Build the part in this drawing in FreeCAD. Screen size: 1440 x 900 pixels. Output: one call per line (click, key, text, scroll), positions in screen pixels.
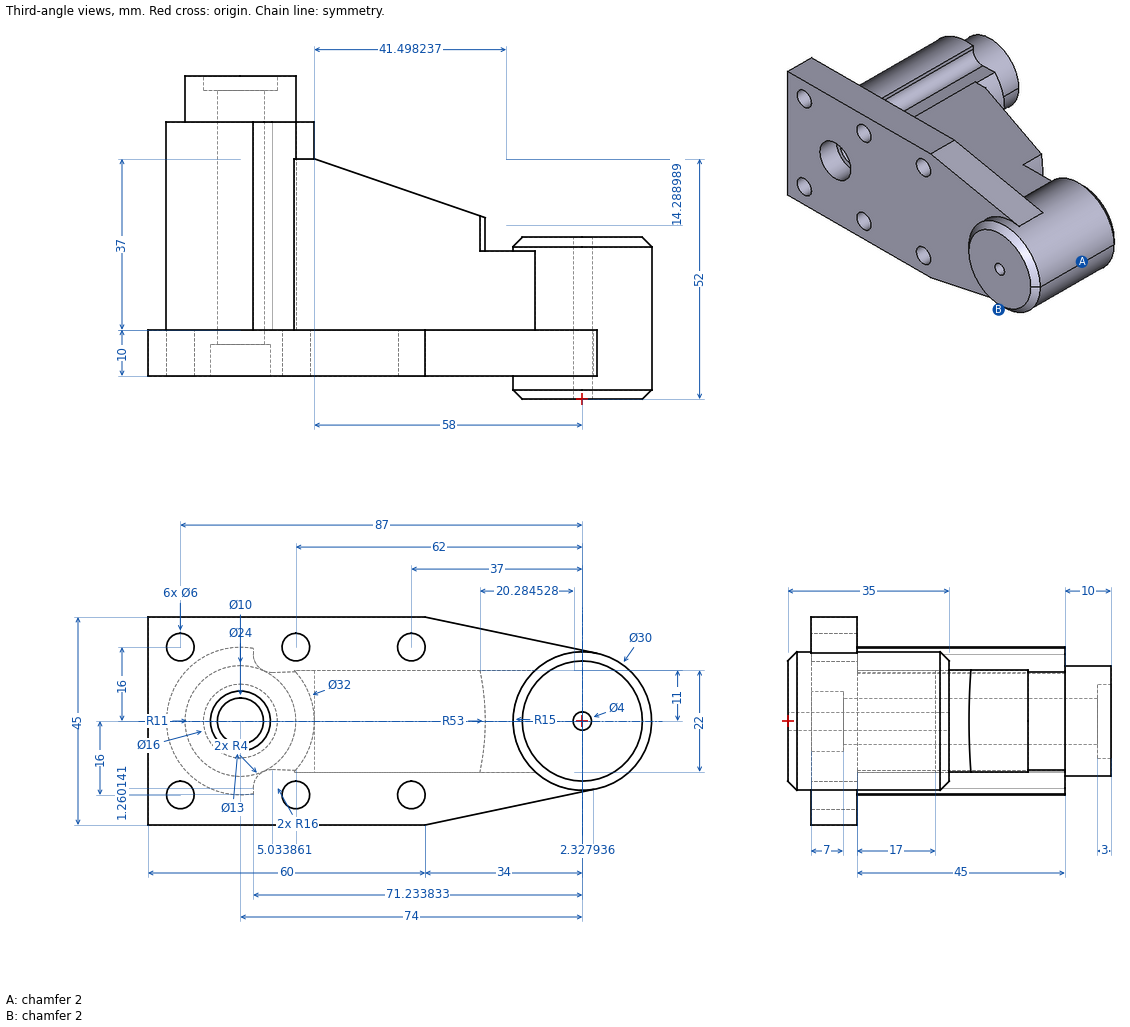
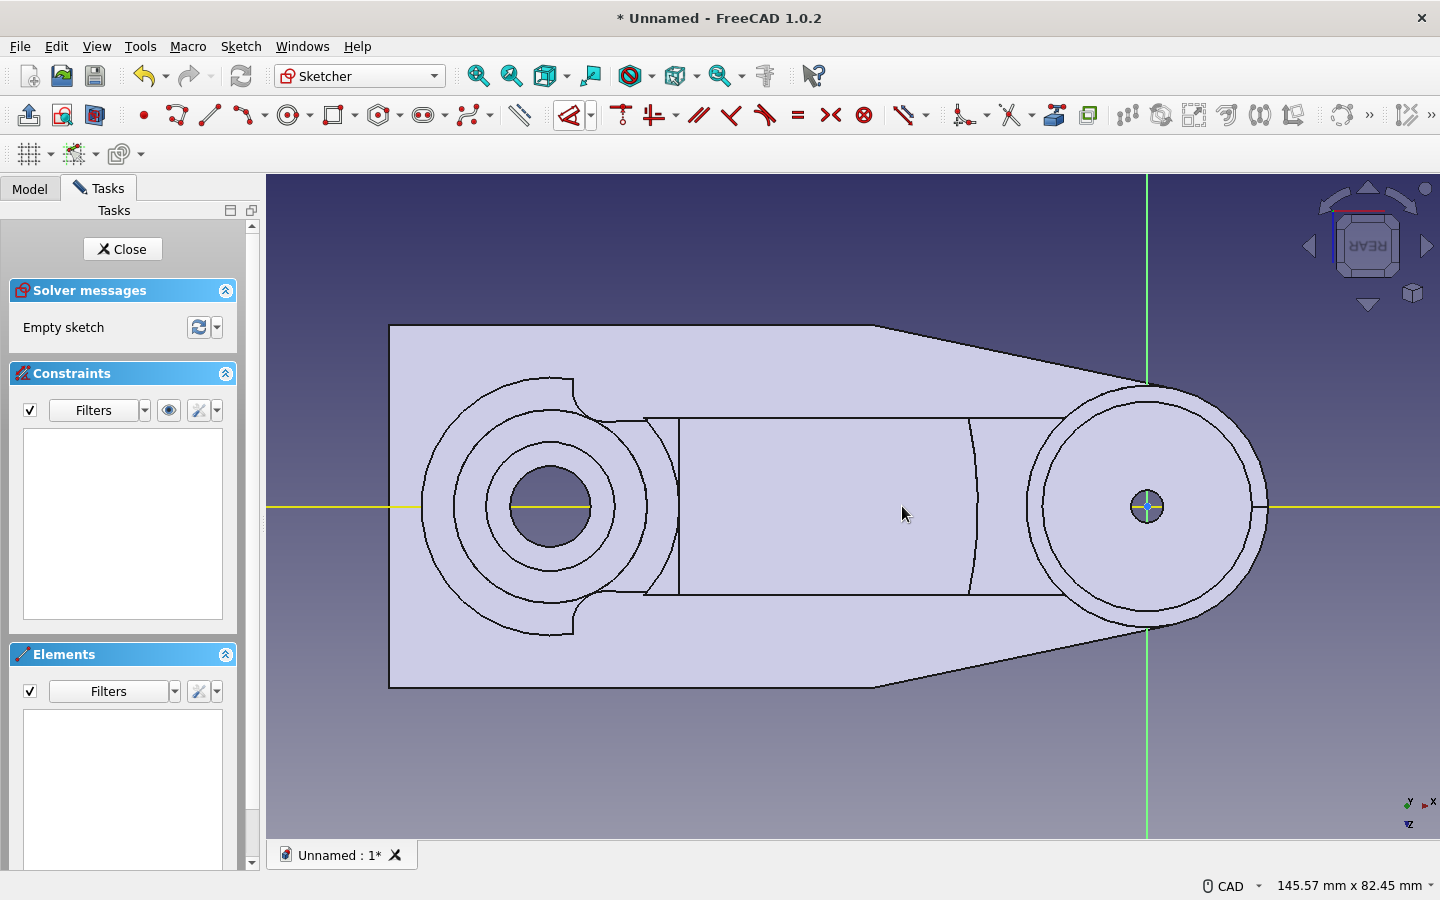
click(288, 116)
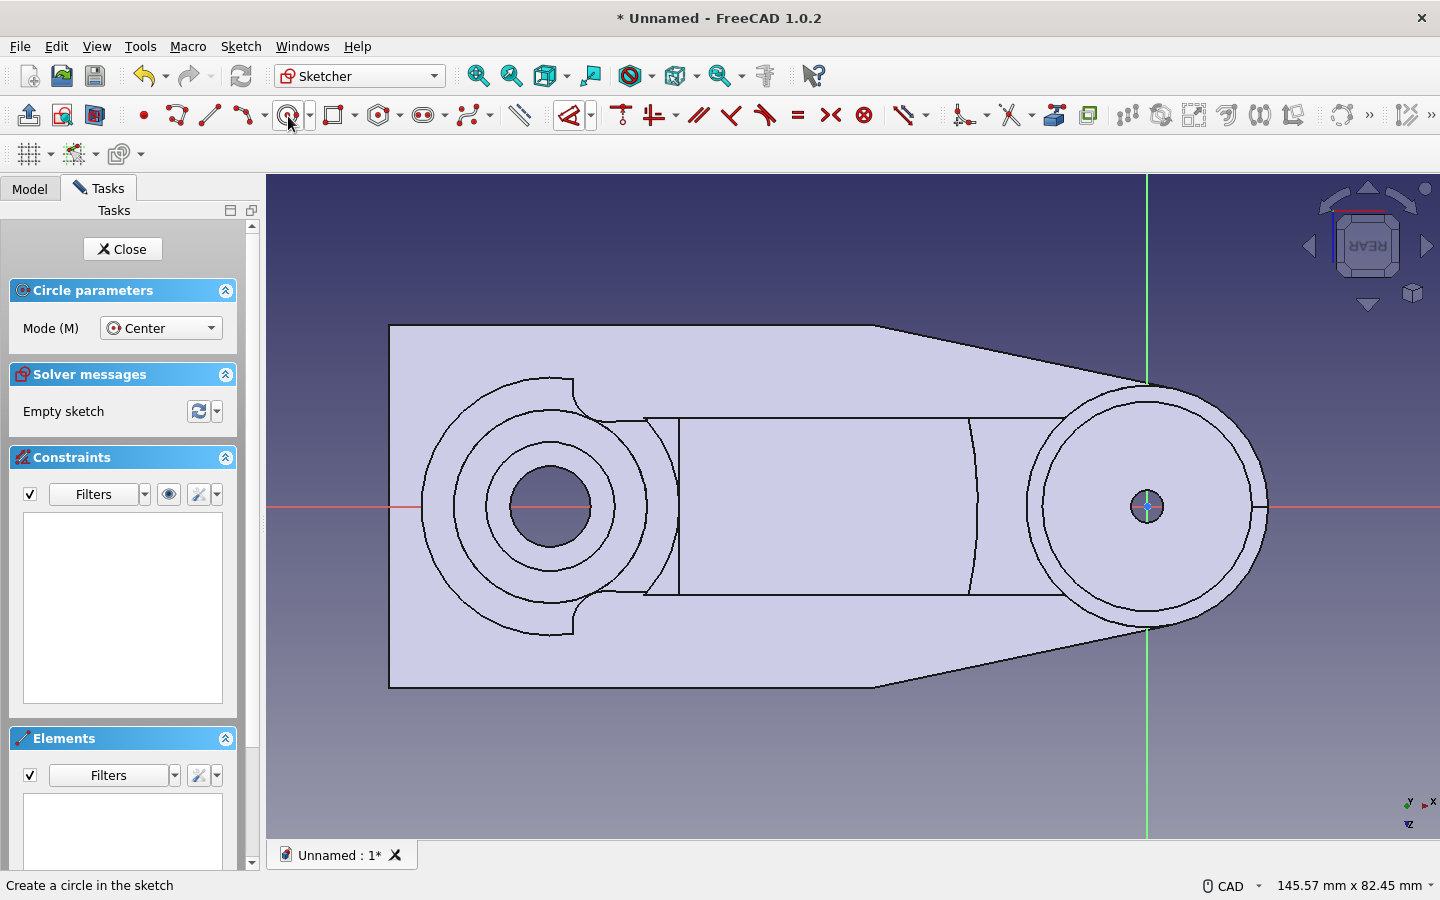
click(446, 636)
click(463, 618)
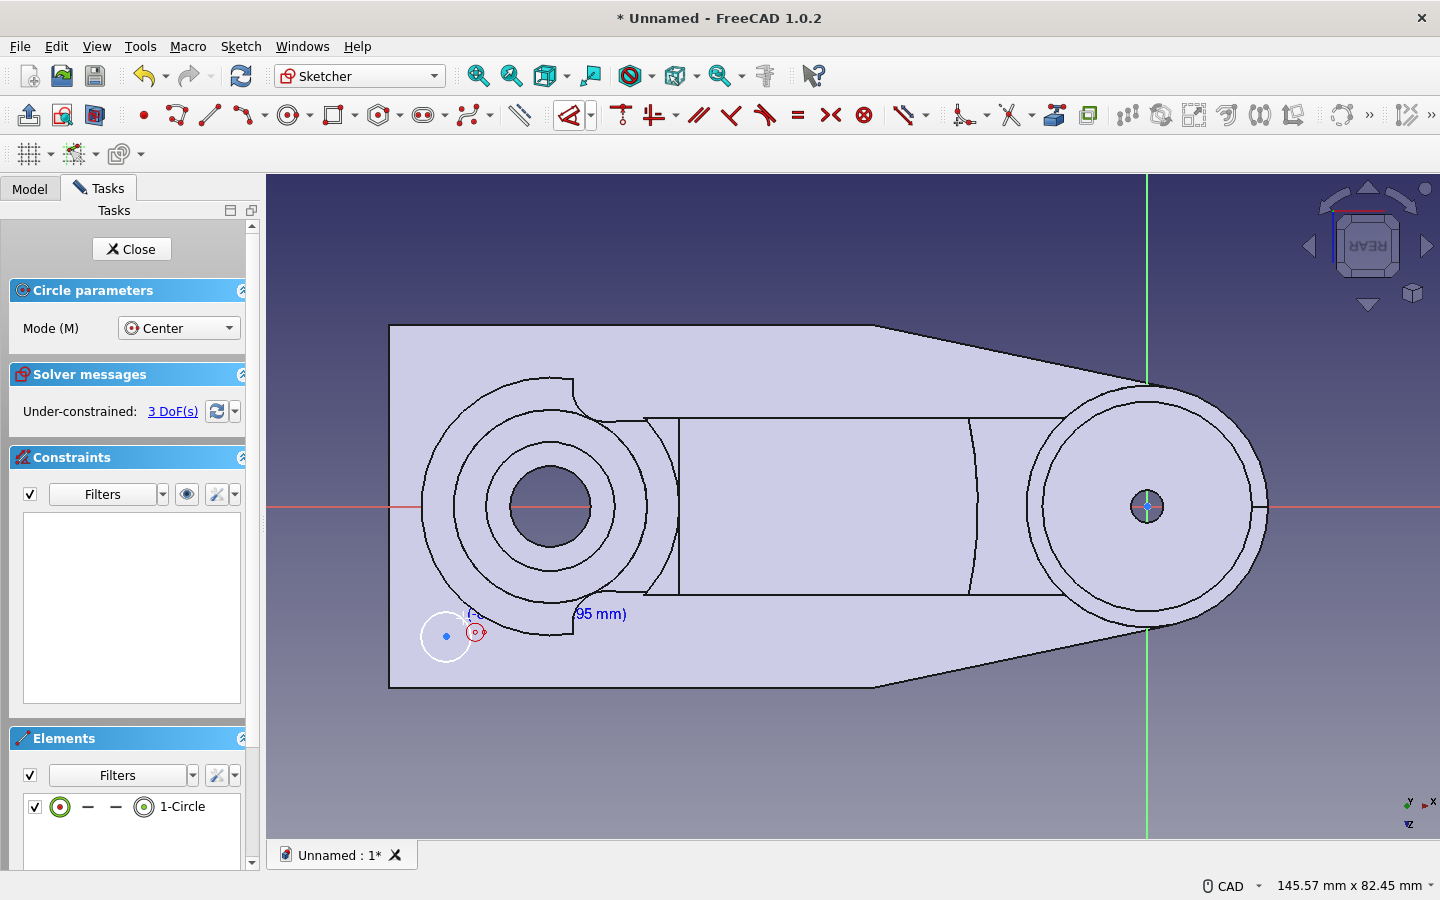
click(647, 636)
click(664, 618)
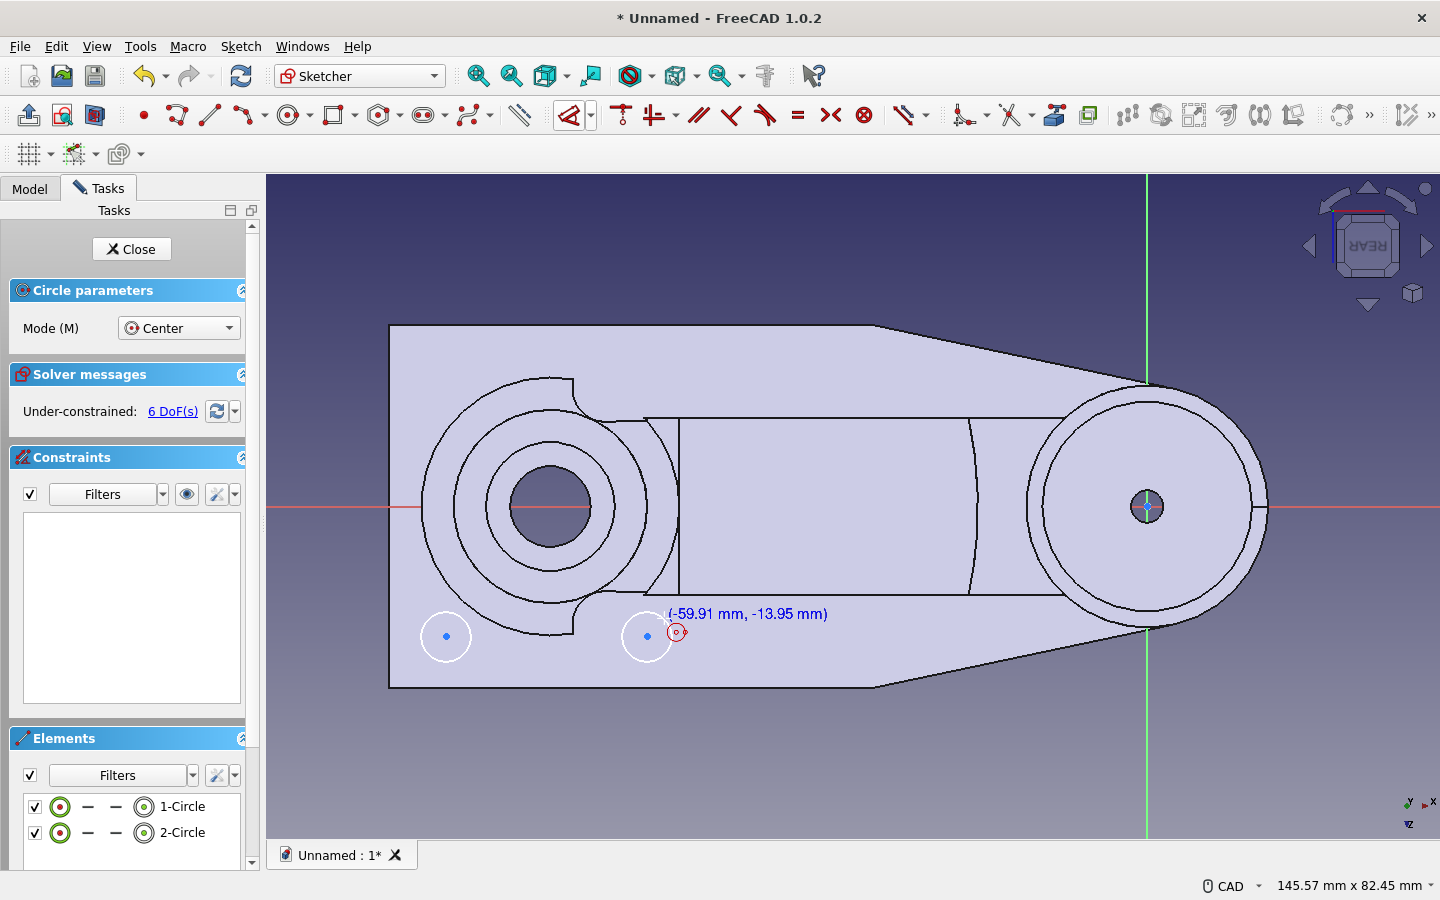
click(849, 636)
click(866, 618)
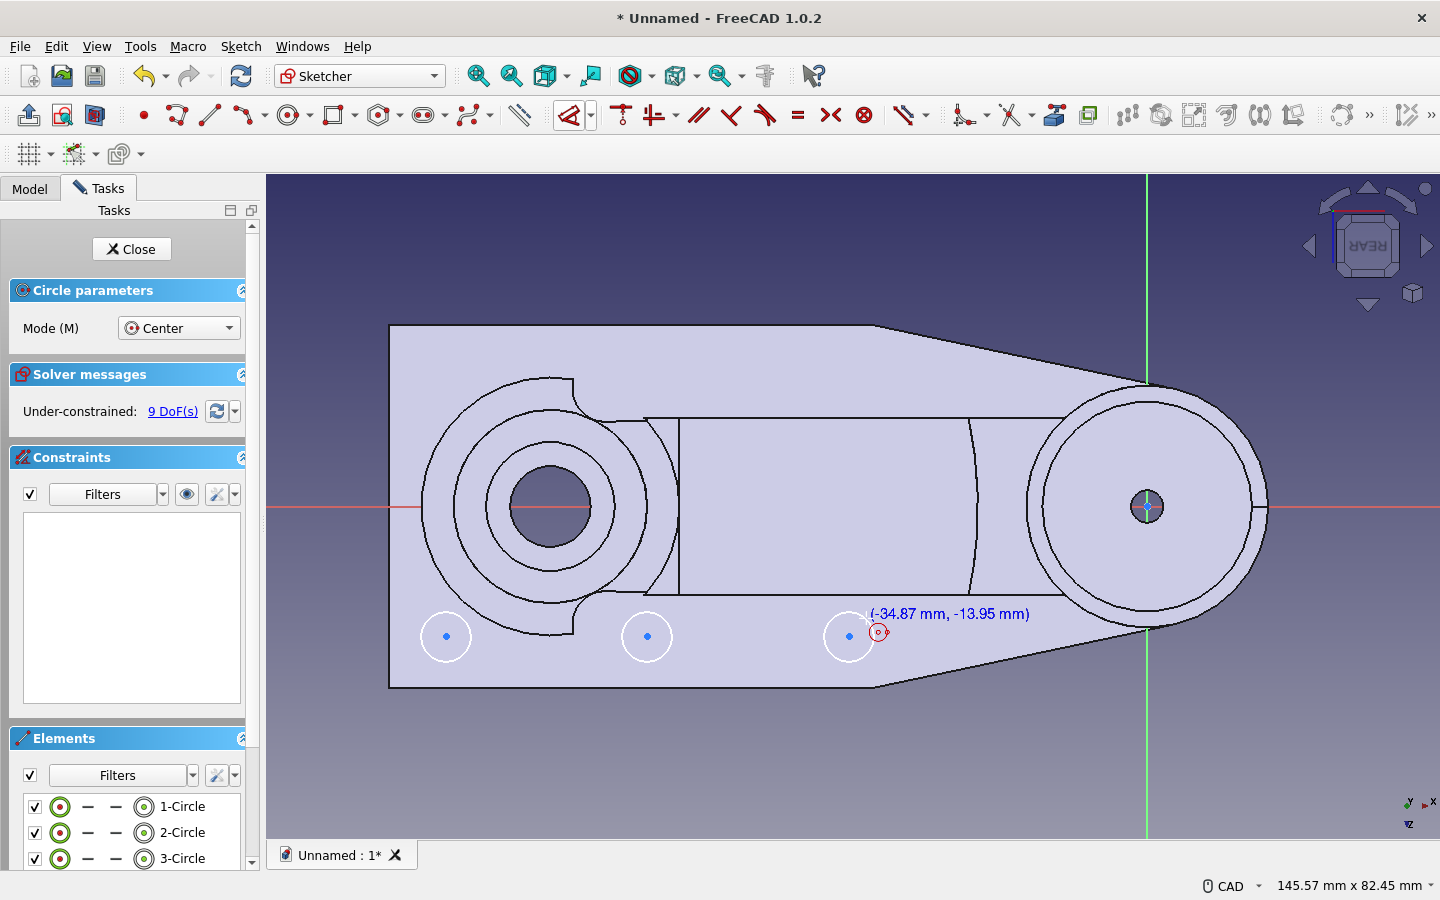
click(446, 377)
click(463, 360)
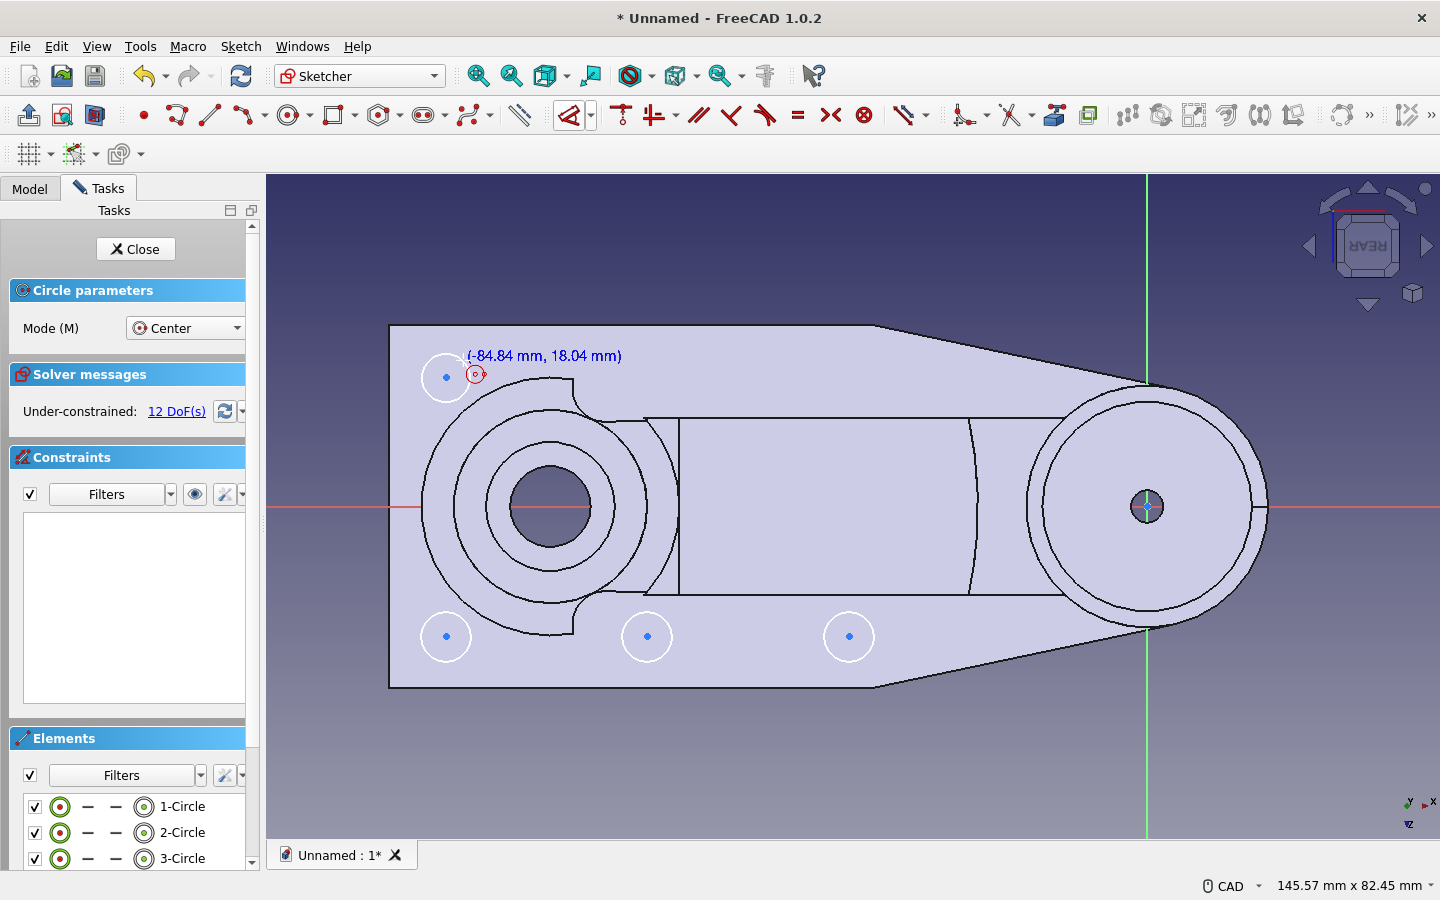
click(849, 377)
click(866, 360)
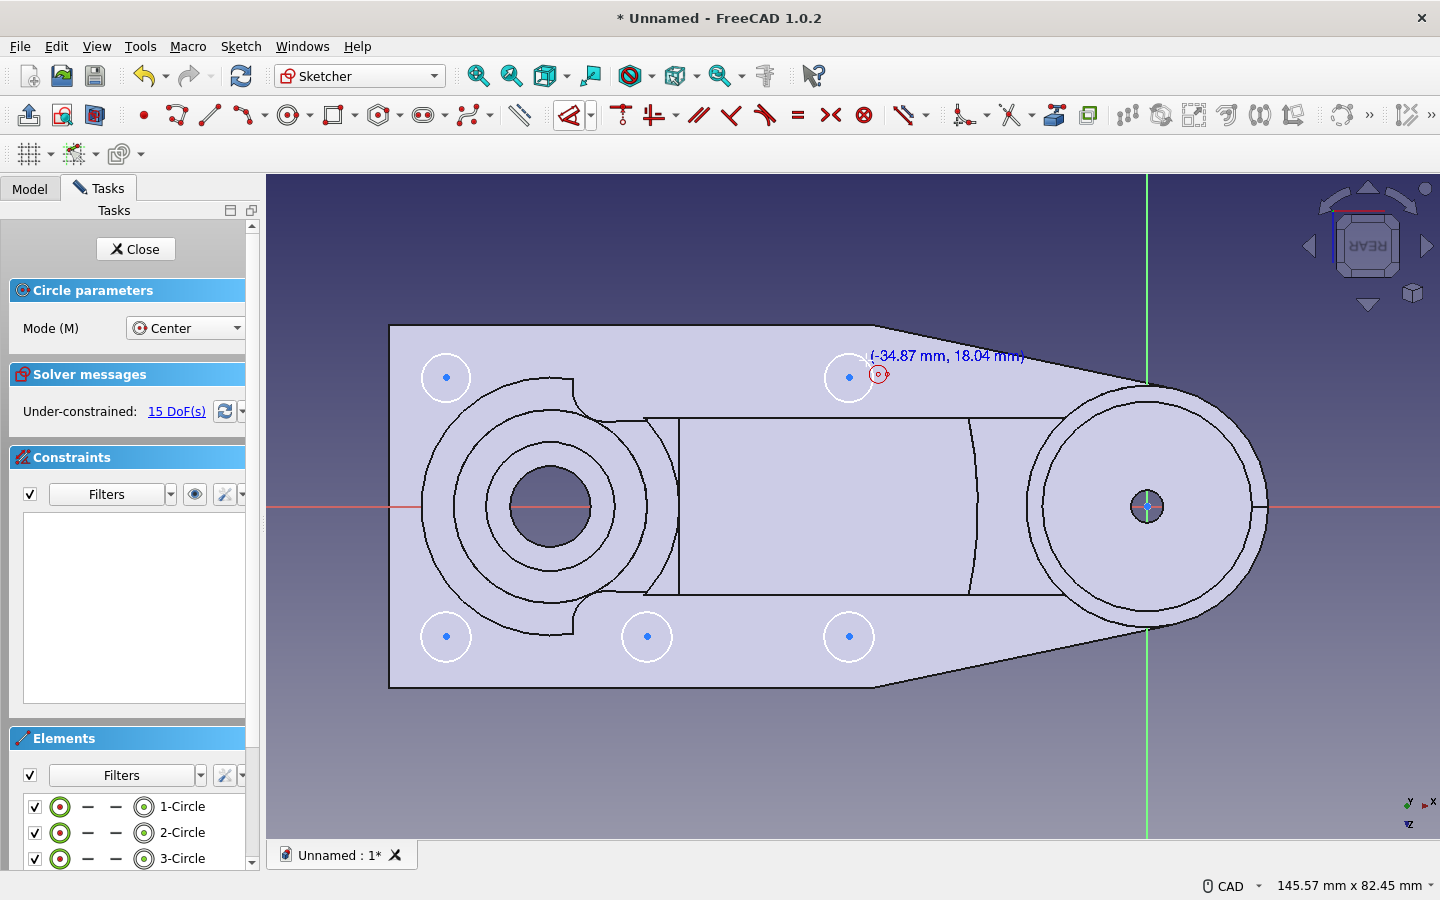
click(647, 377)
click(664, 360)
key(Escape)